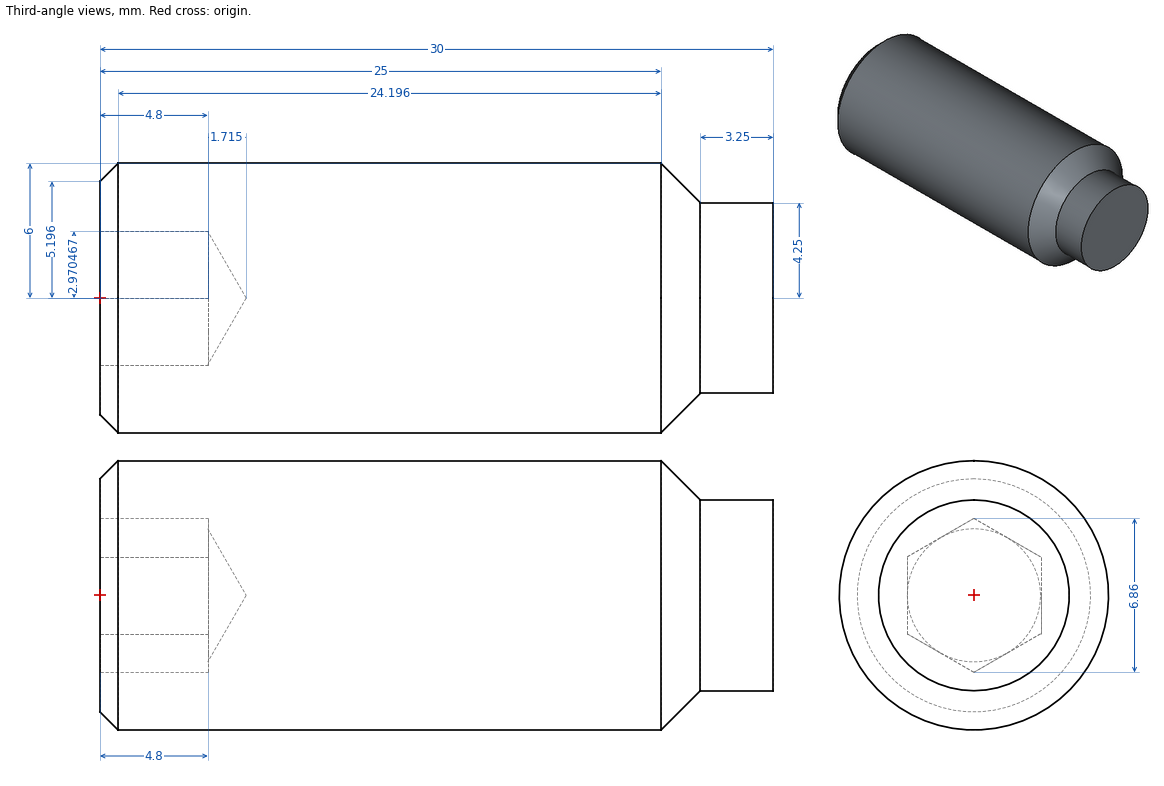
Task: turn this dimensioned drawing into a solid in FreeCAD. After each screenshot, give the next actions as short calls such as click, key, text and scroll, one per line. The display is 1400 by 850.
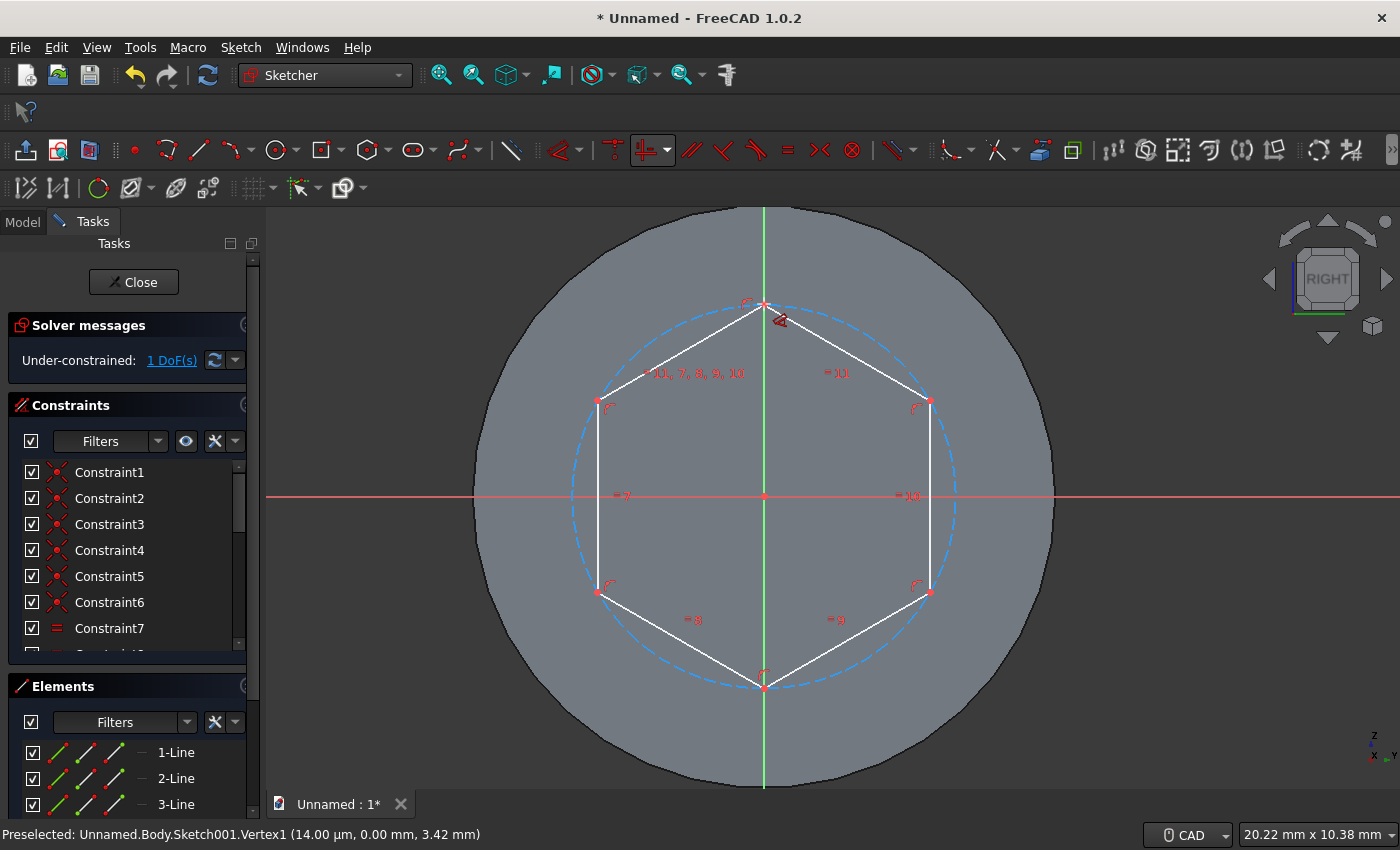
click(764, 689)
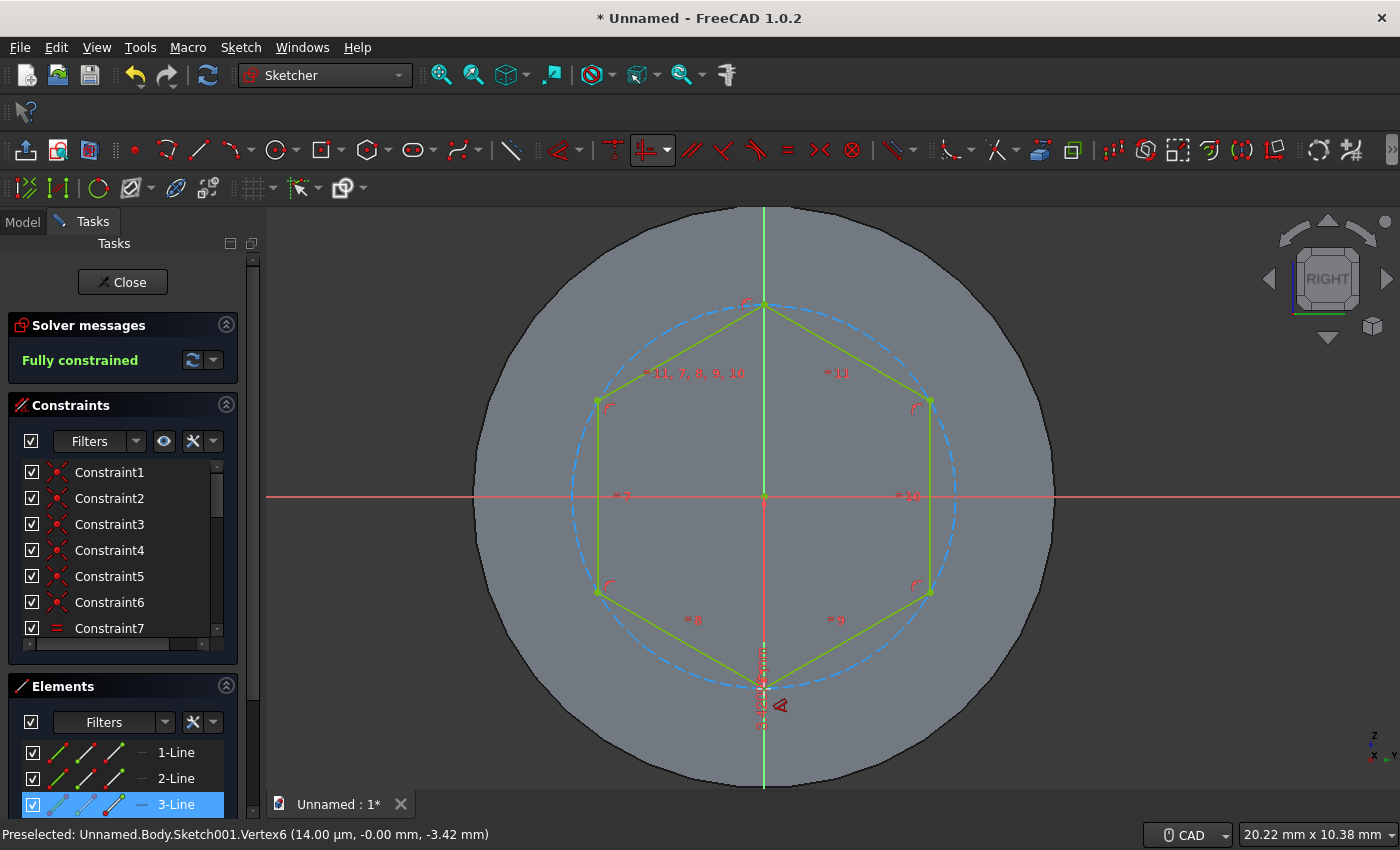
click(764, 305)
click(798, 409)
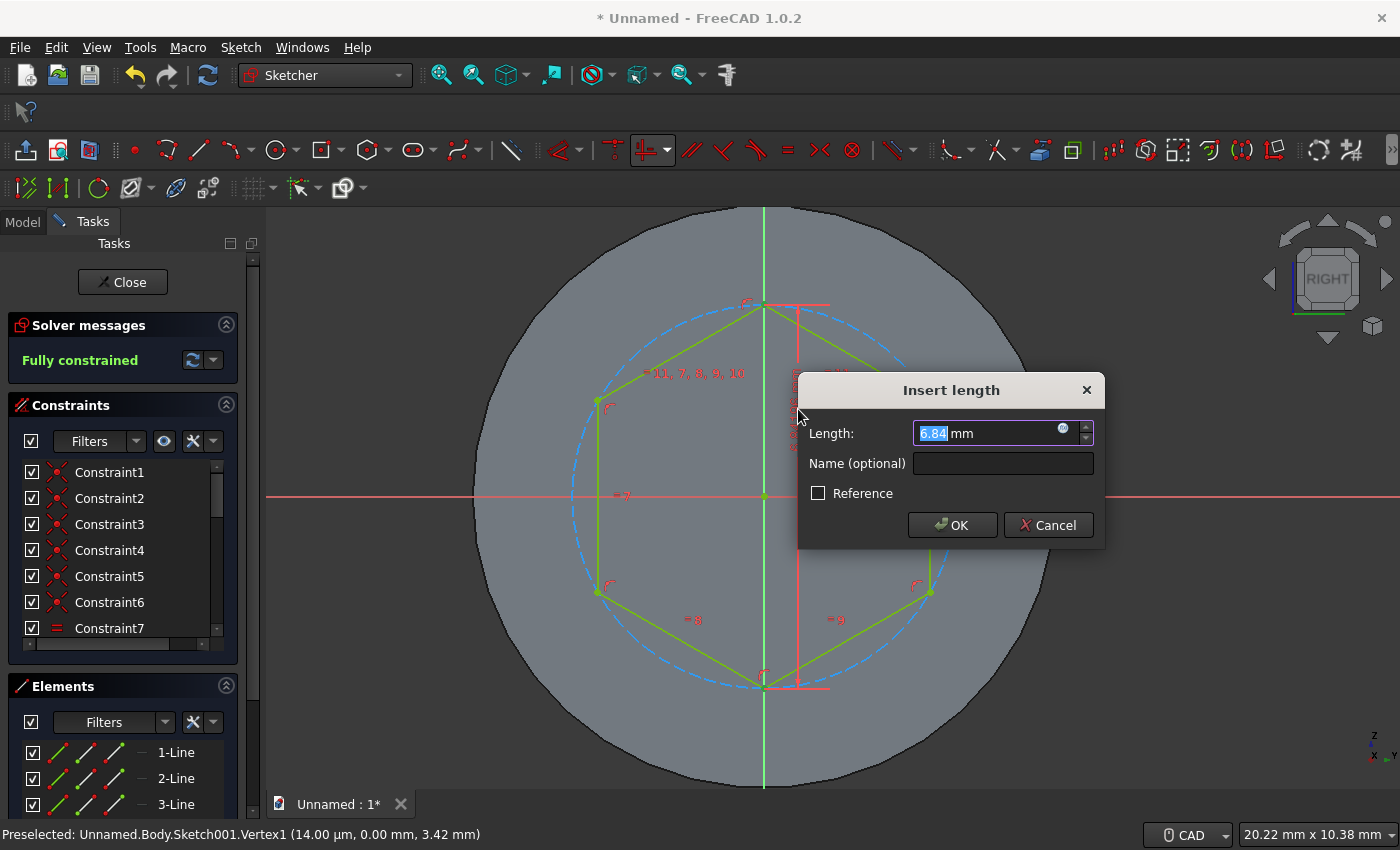
text(6.86)
key(Return)
key(Escape)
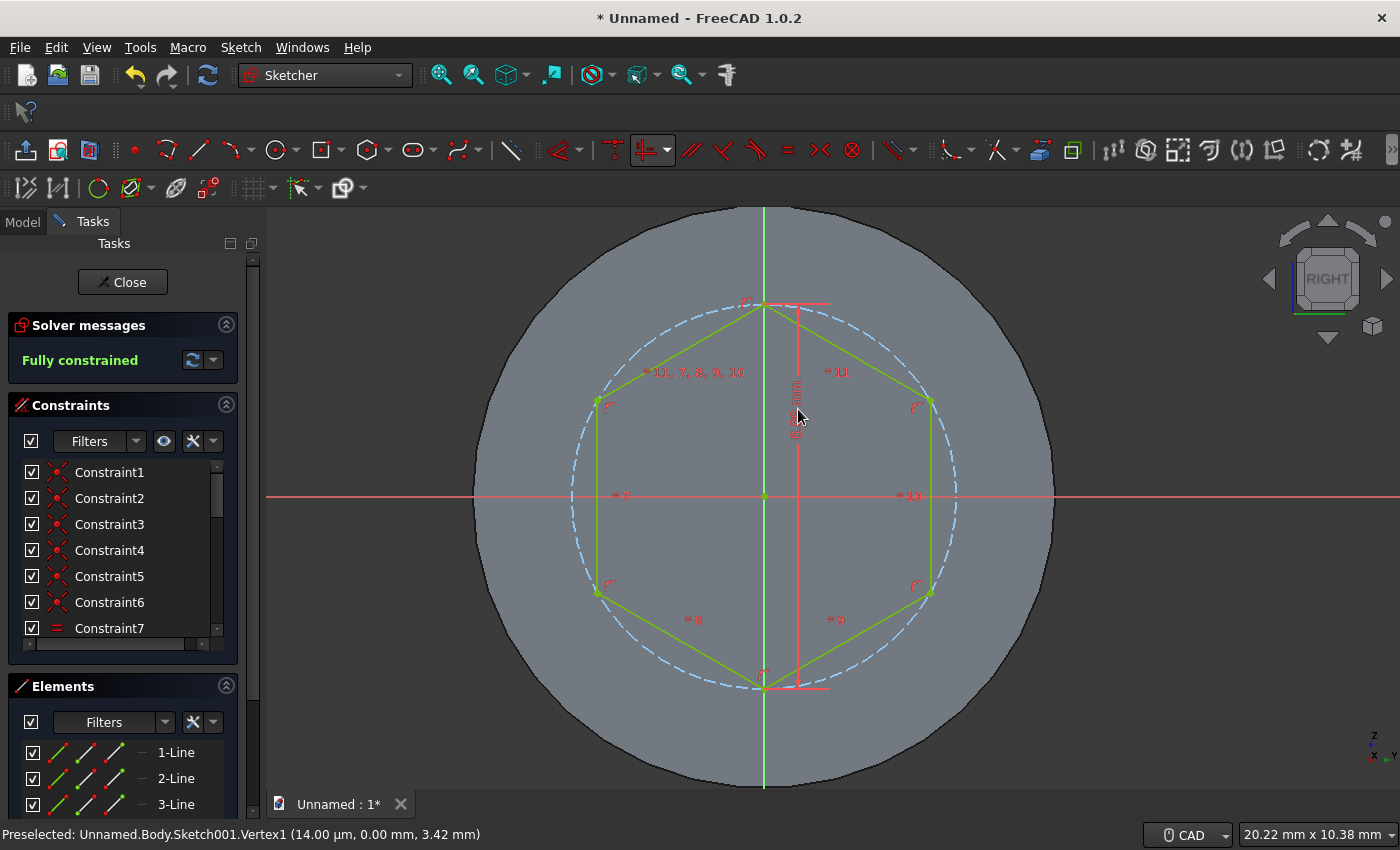
click(123, 282)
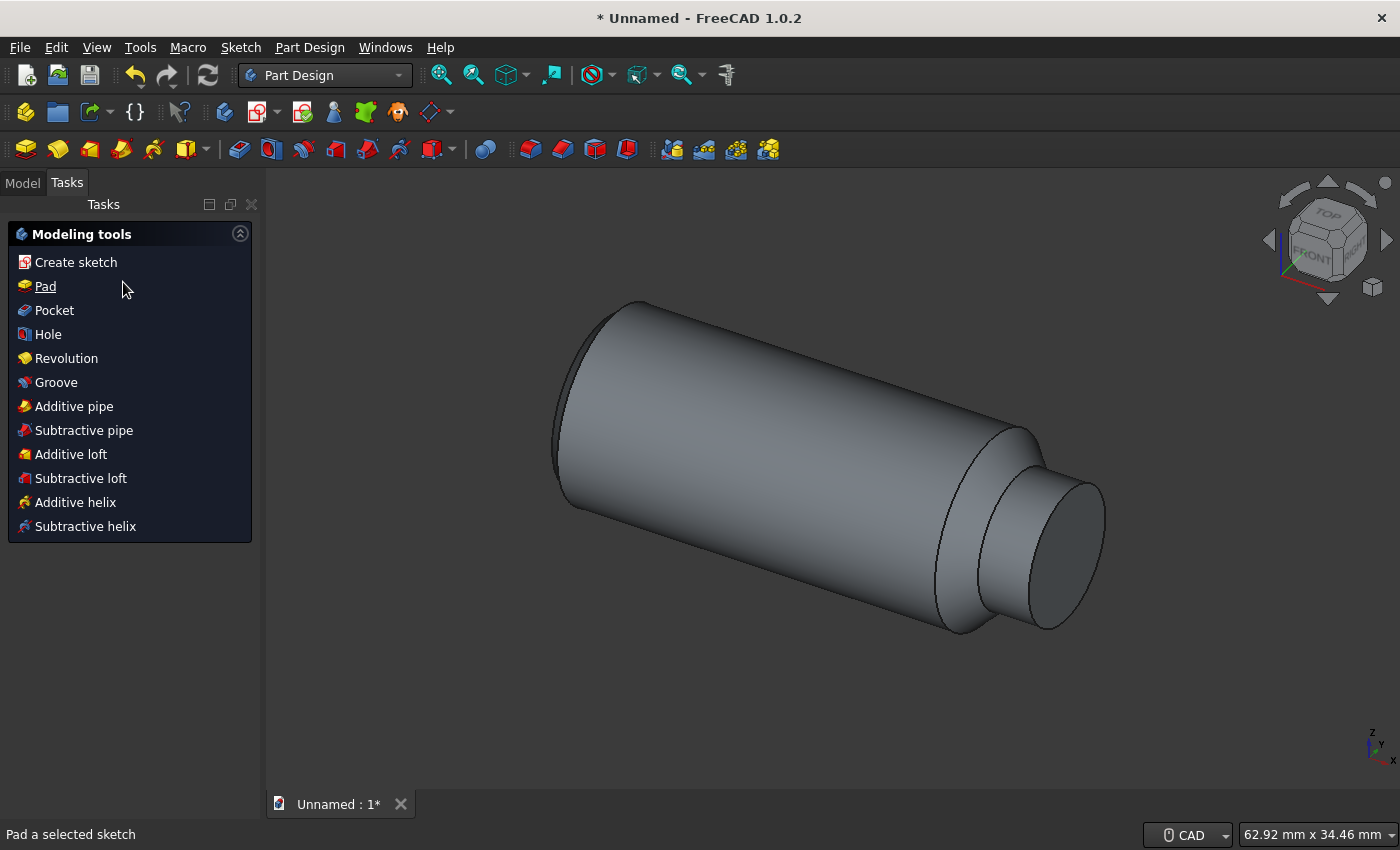
click(240, 150)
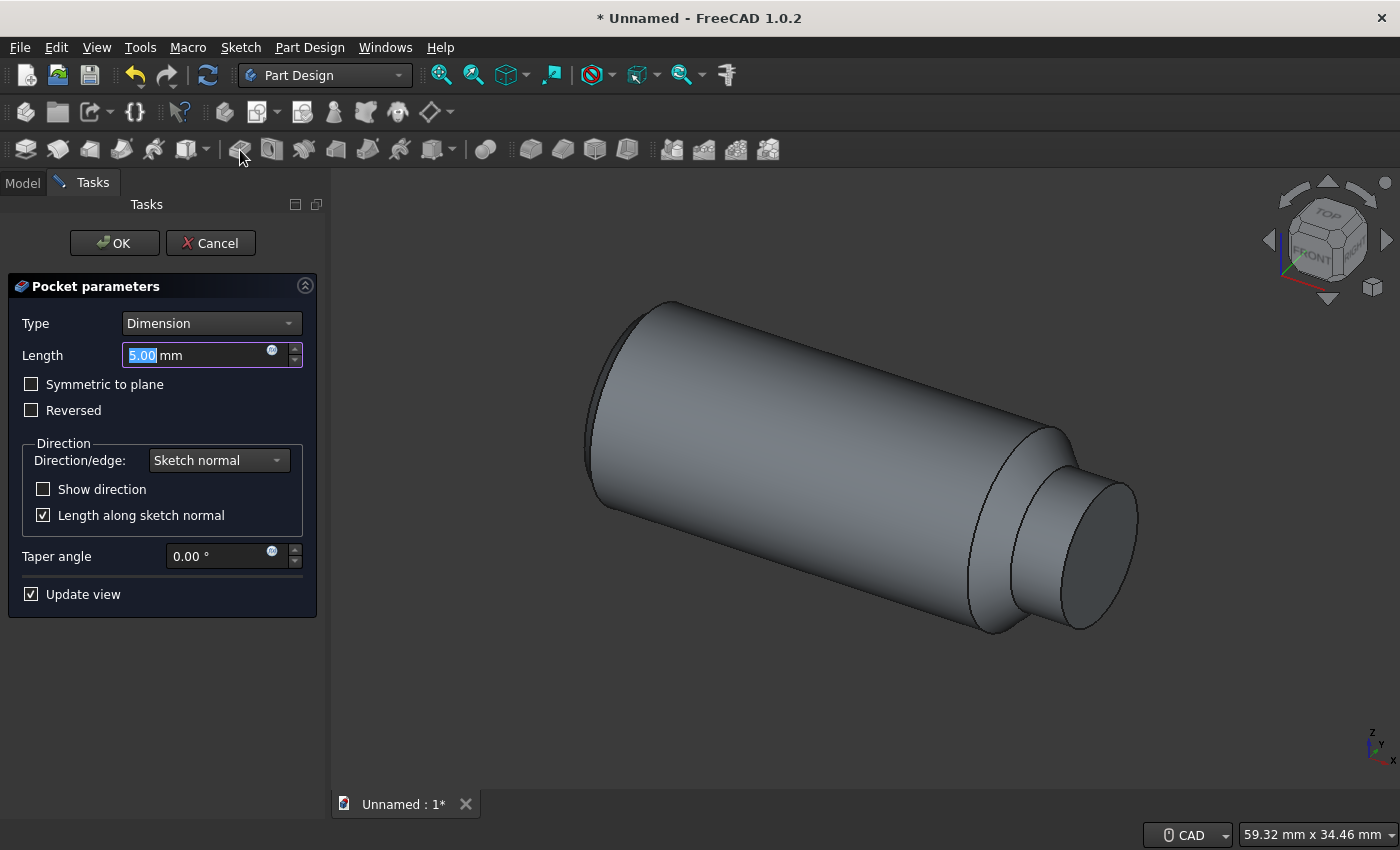
text(4.8)
key(Tab)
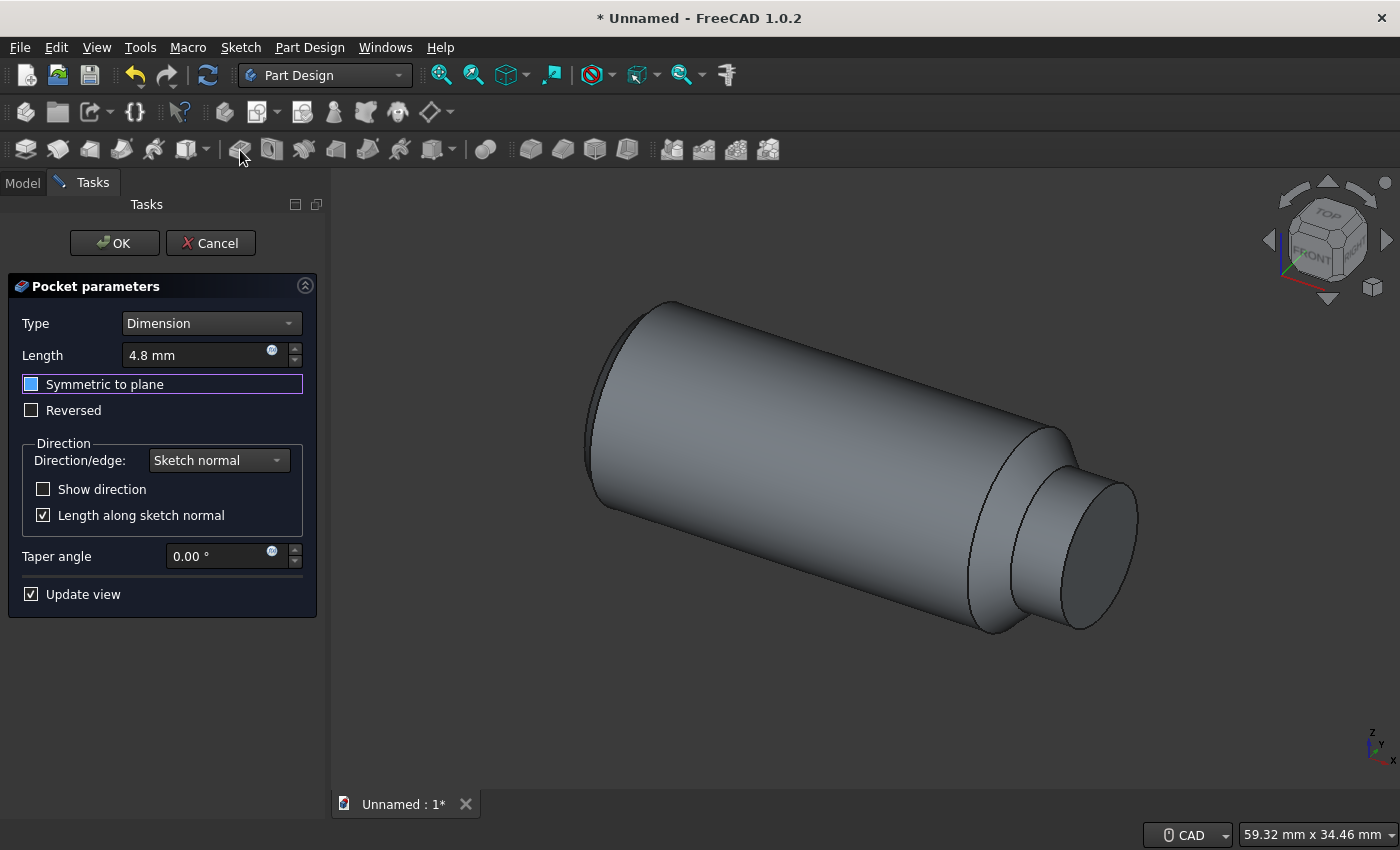
click(30, 410)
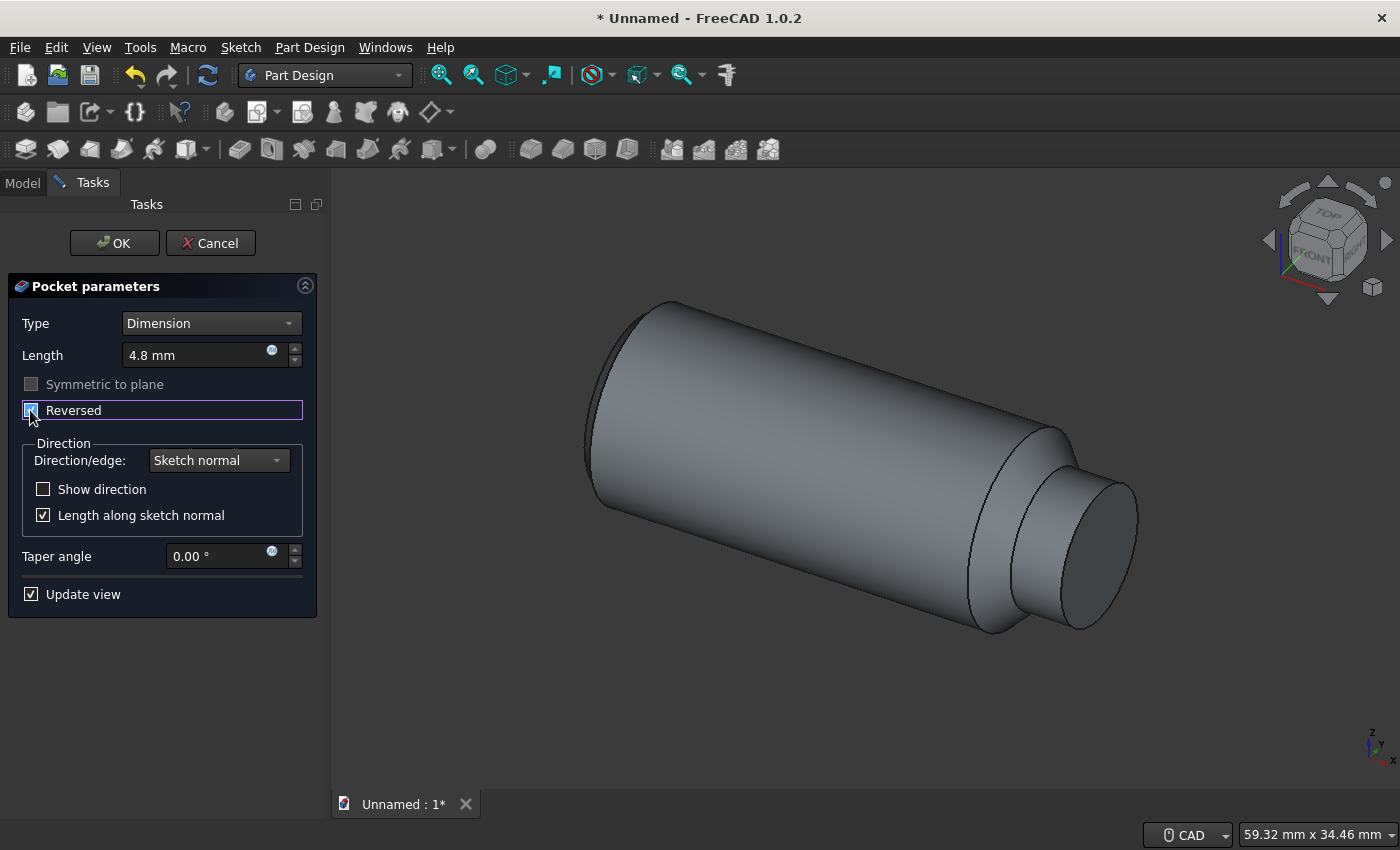
click(115, 243)